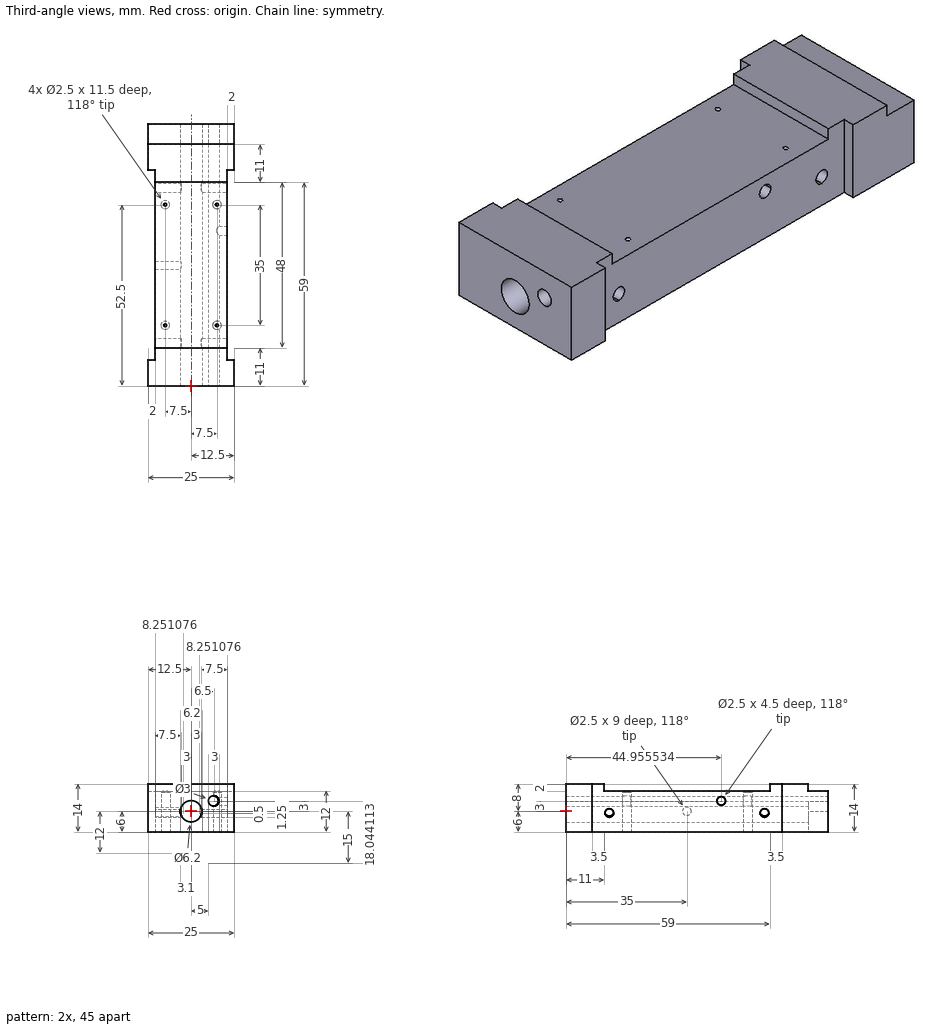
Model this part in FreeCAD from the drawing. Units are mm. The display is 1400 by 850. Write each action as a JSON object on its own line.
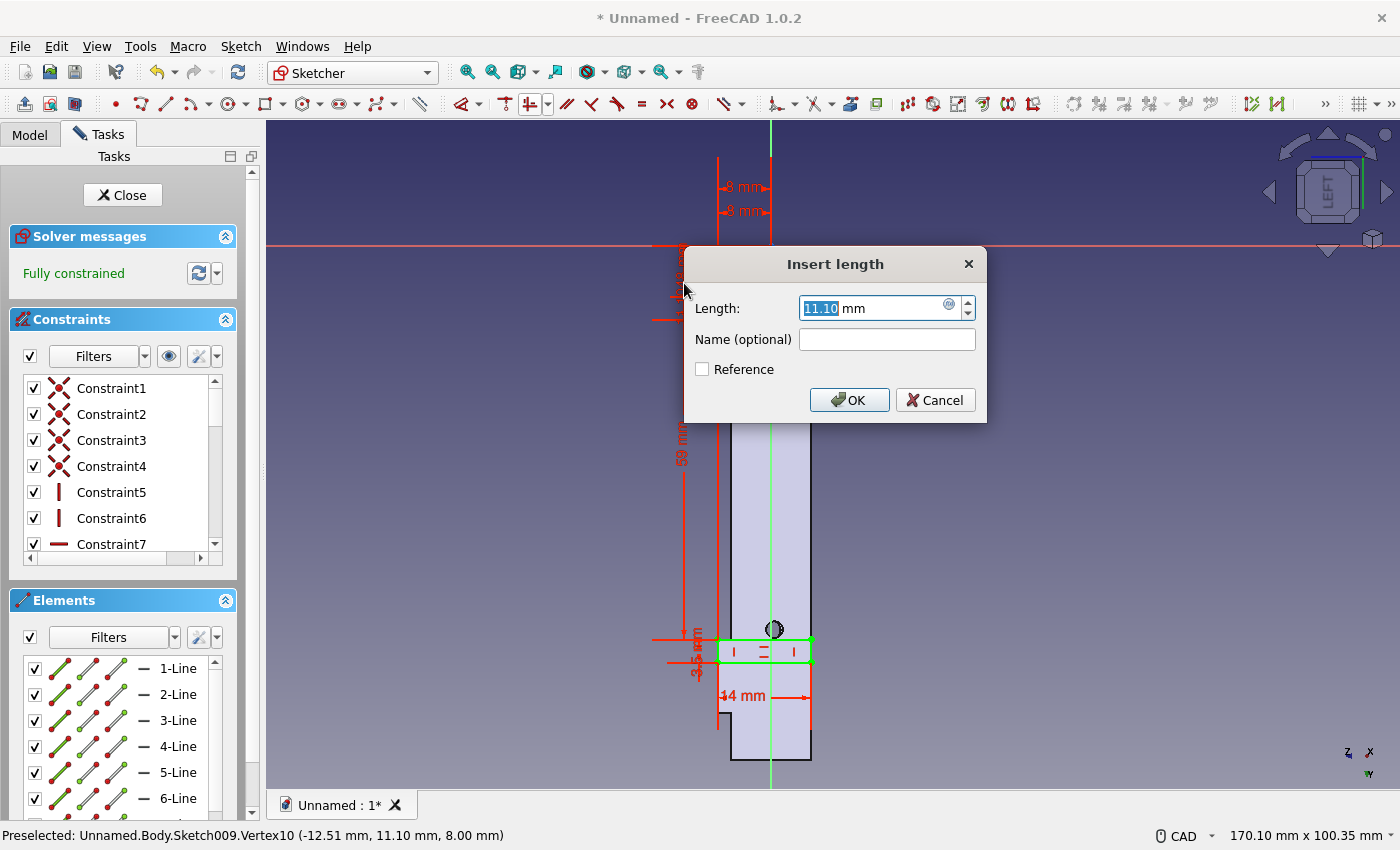
{"action": "type", "text": "11"}
{"action": "key", "text": "Return"}
{"action": "key", "text": "Escape"}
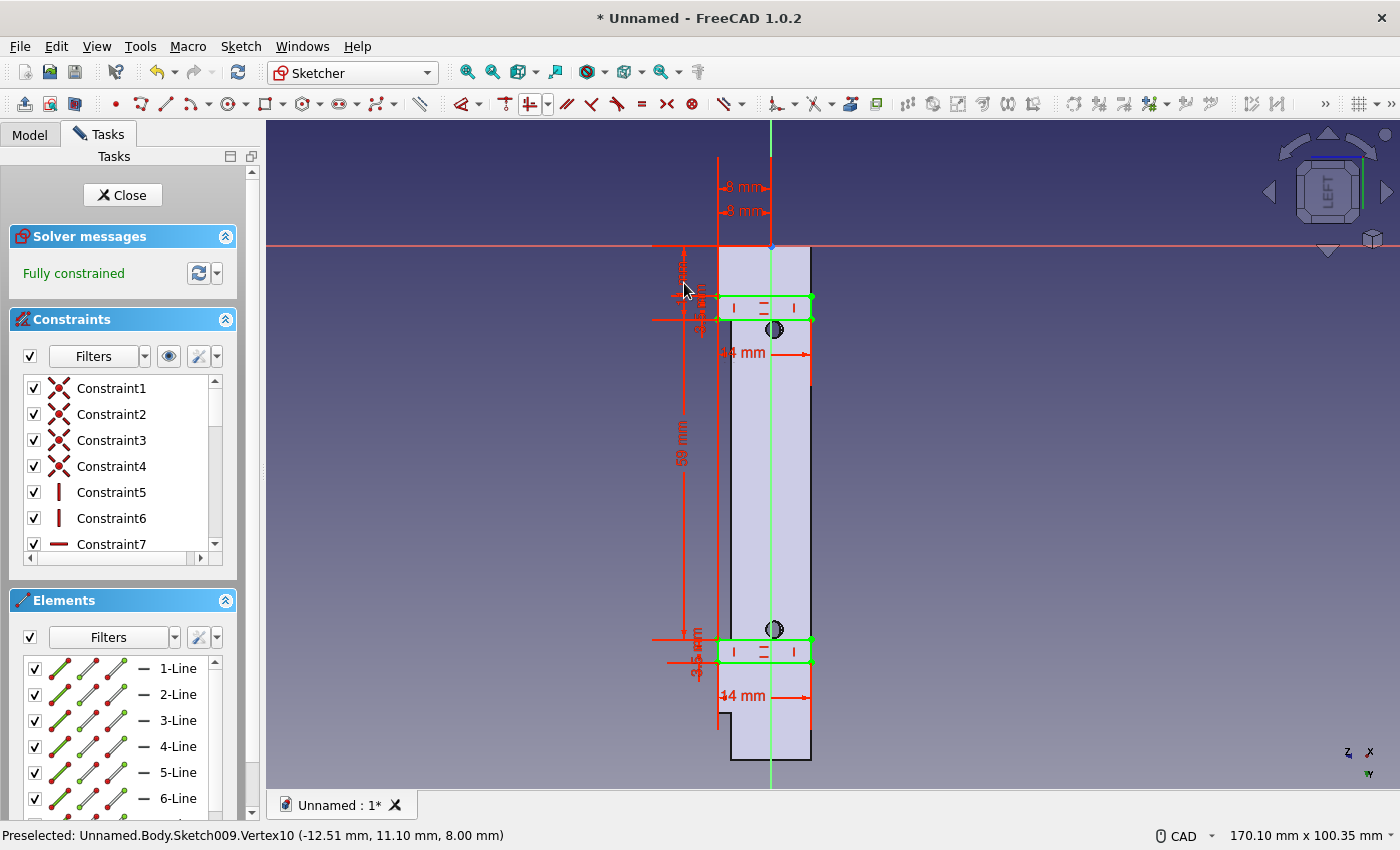
{"action": "left_click", "coordinate": [123, 195]}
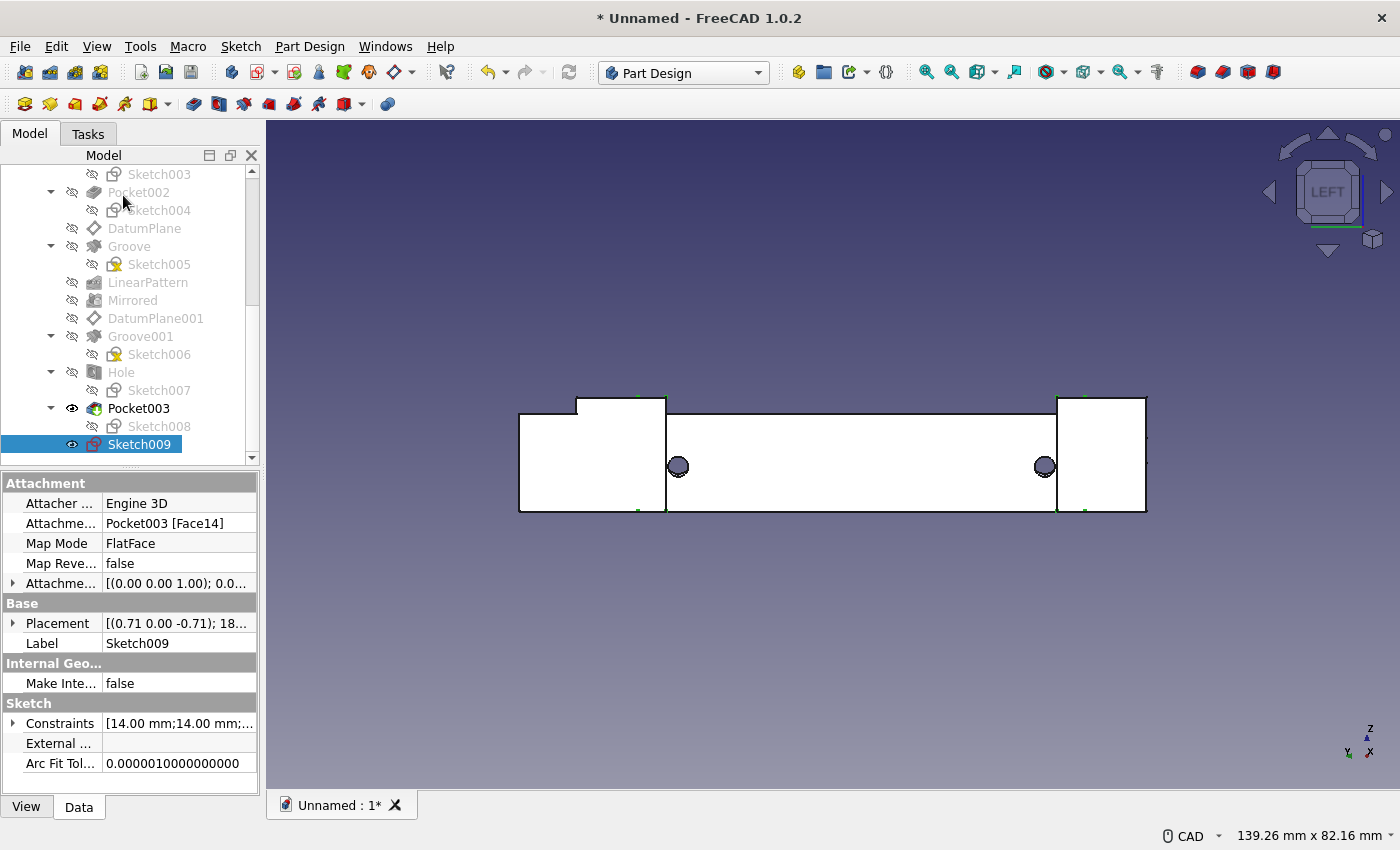
{"action": "left_click", "coordinate": [194, 104]}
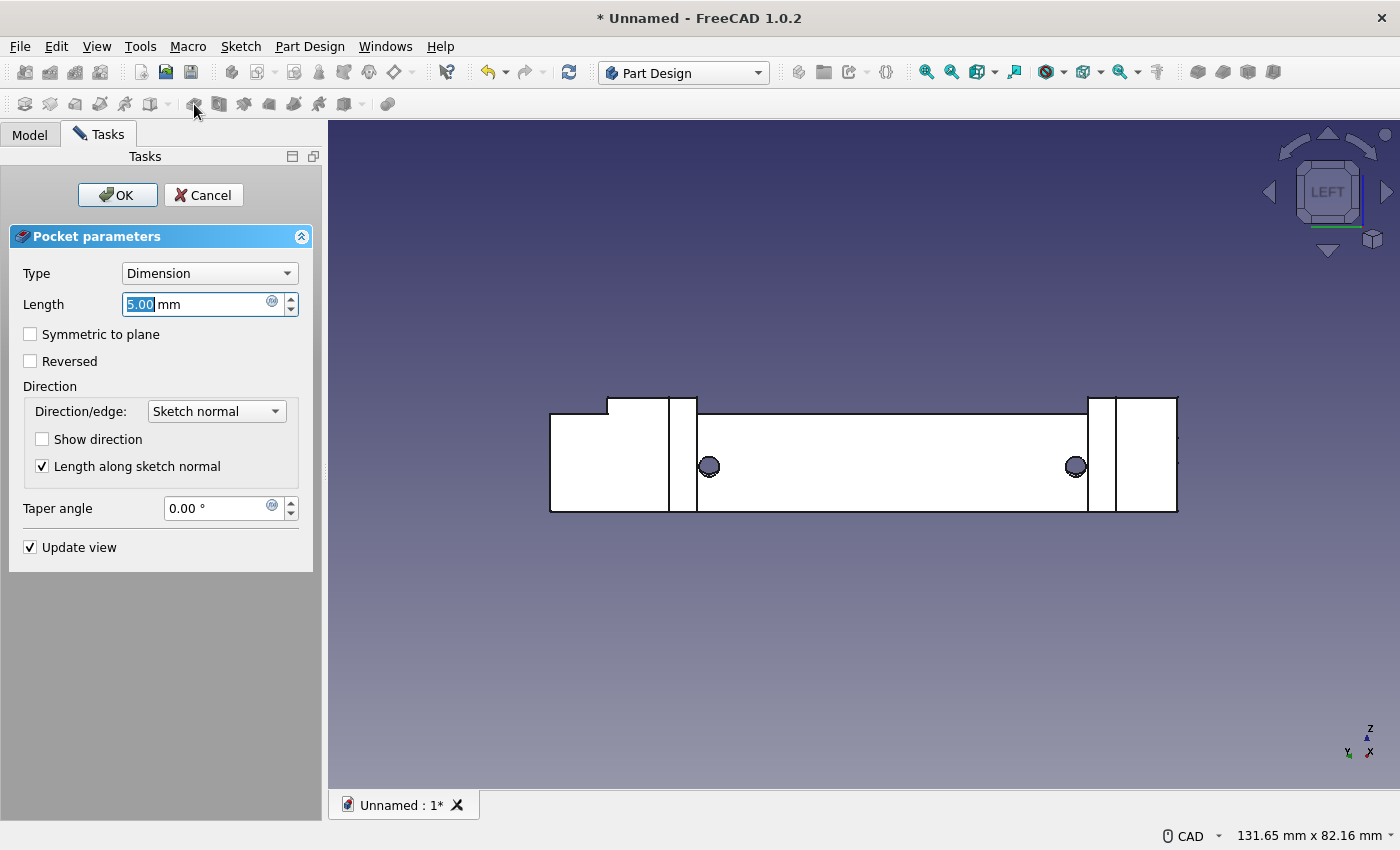
{"action": "type", "text": "2"}
{"action": "key", "text": "Tab"}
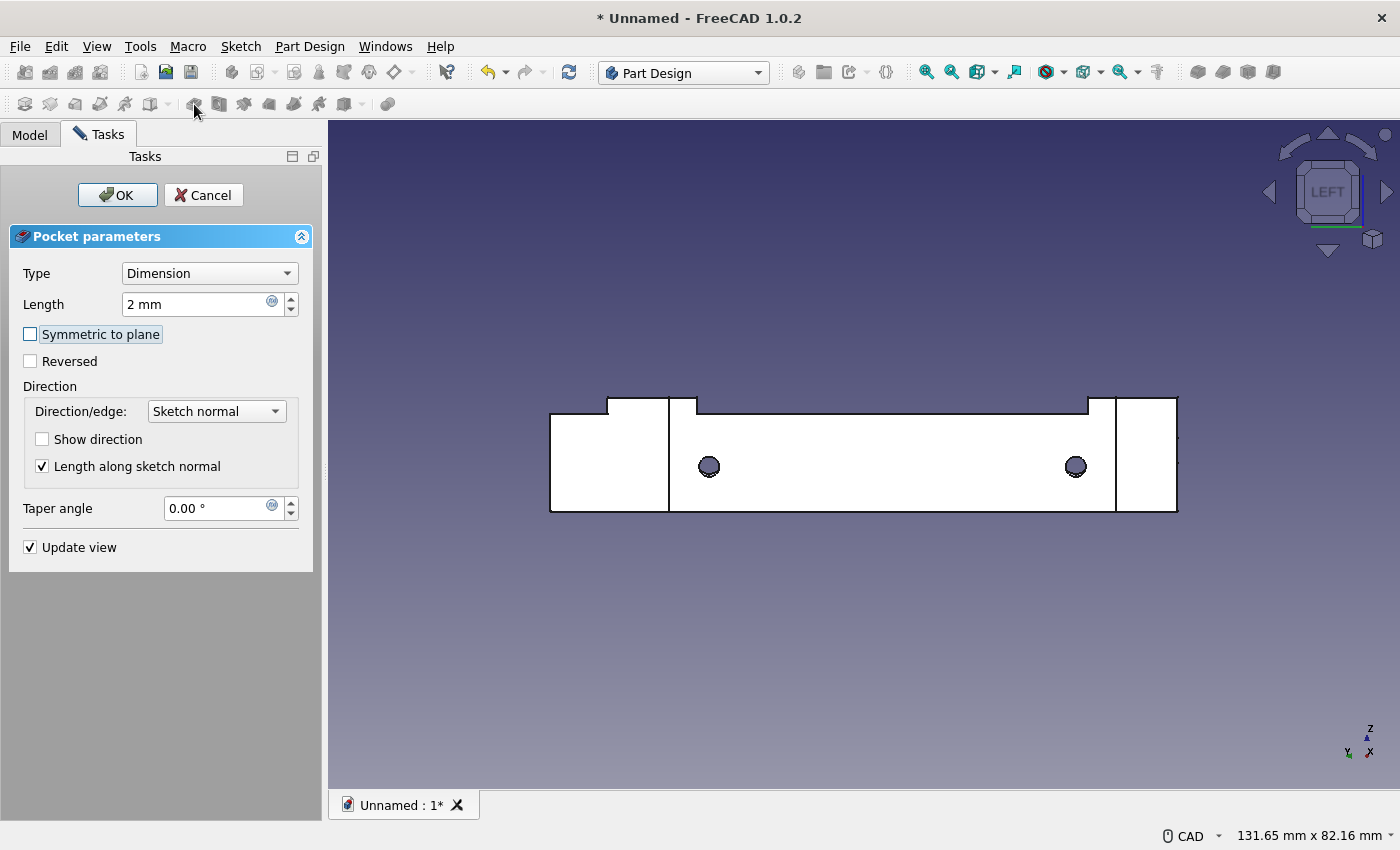
{"action": "left_click", "coordinate": [118, 195]}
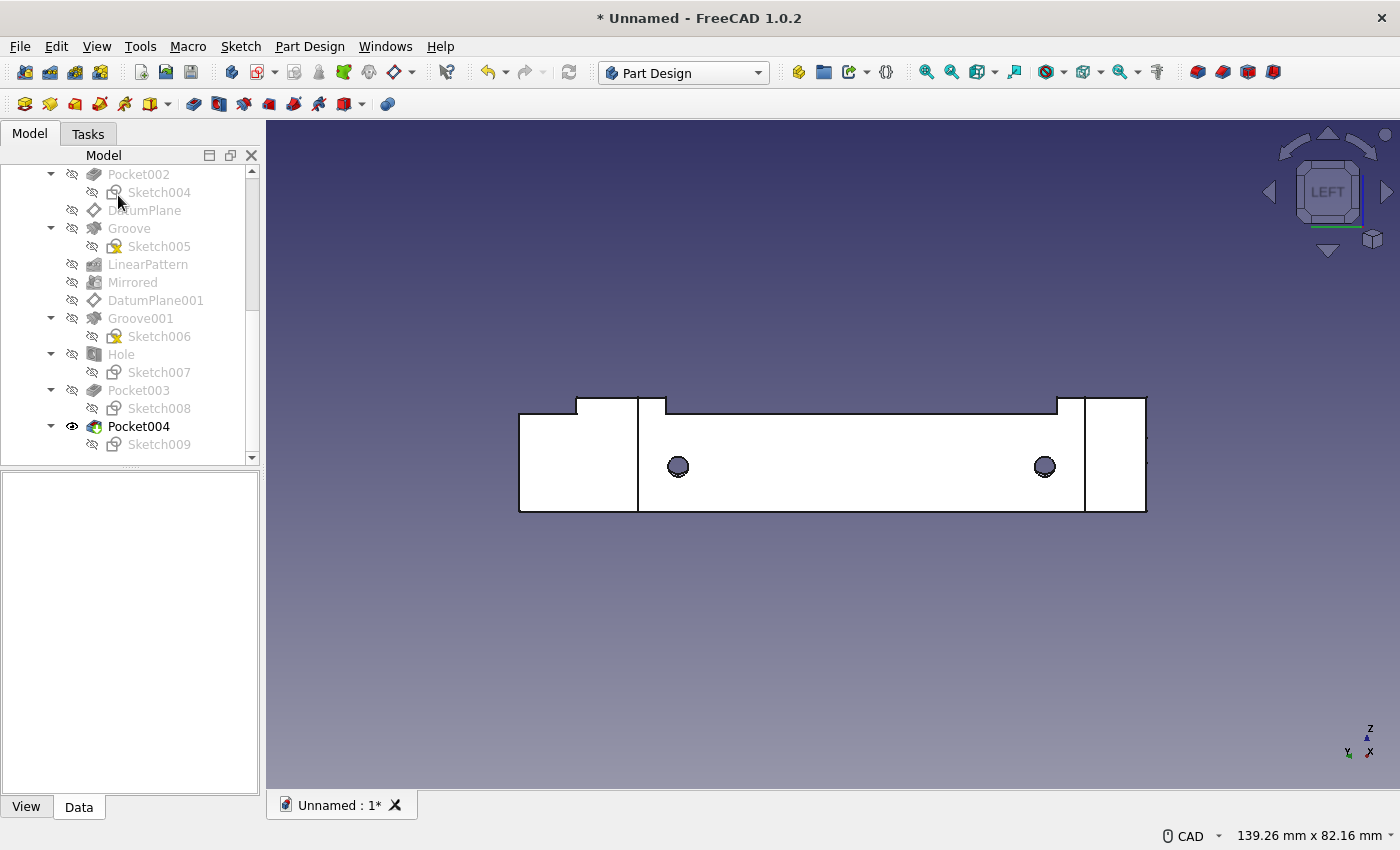
{"action": "key", "text": "0"}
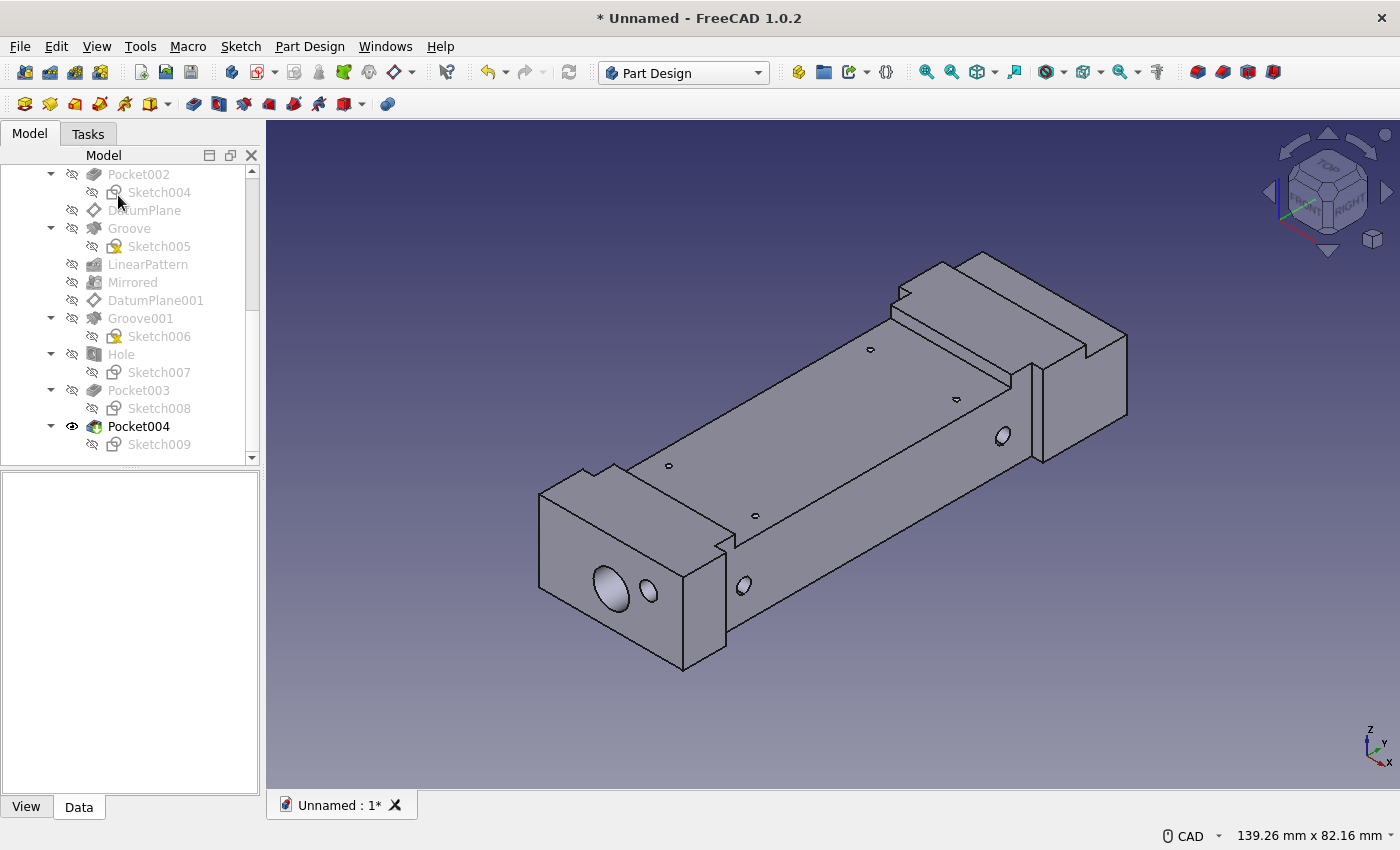
{"action": "left_click", "coordinate": [783, 552]}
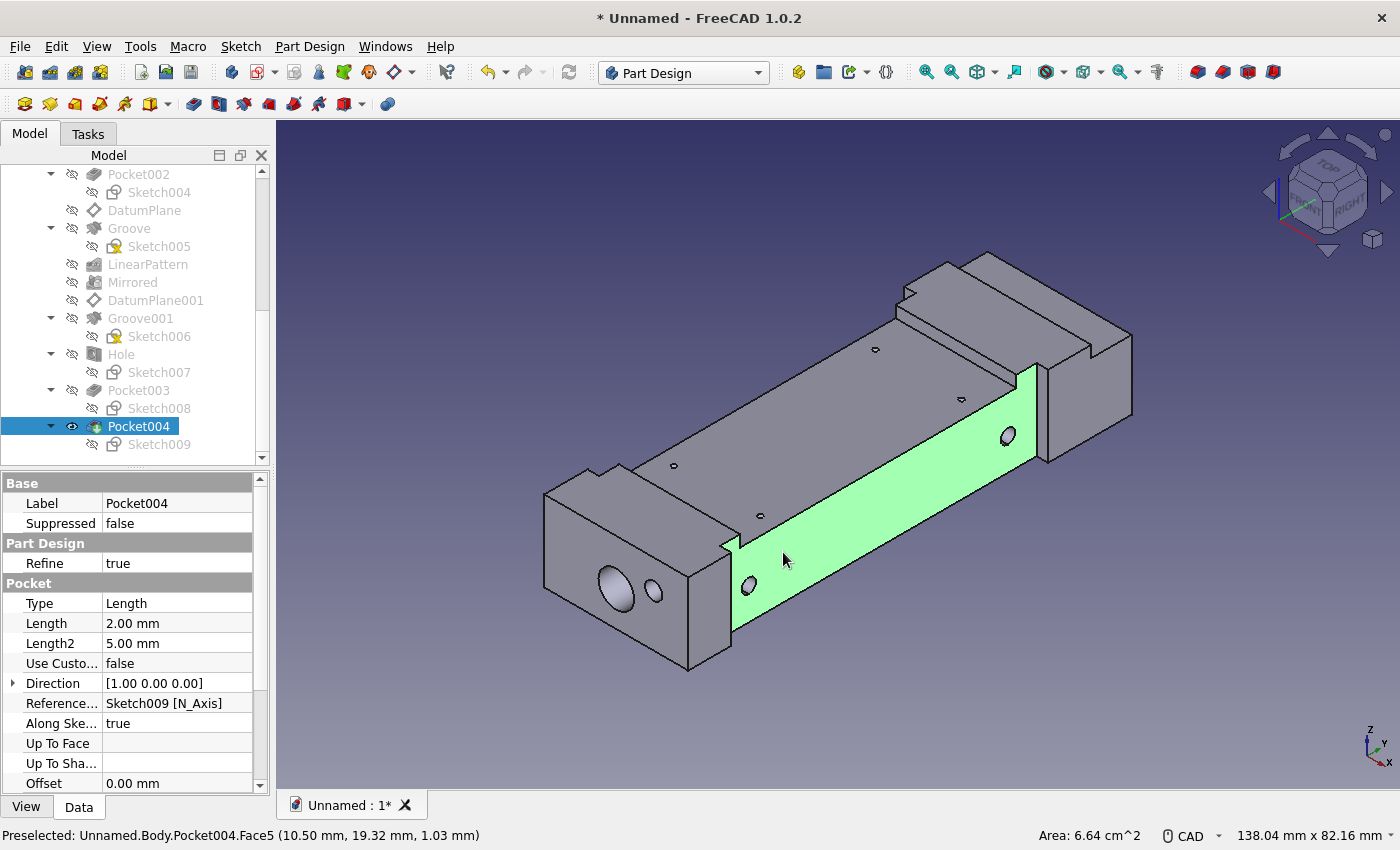
{"action": "left_click", "coordinate": [256, 72]}